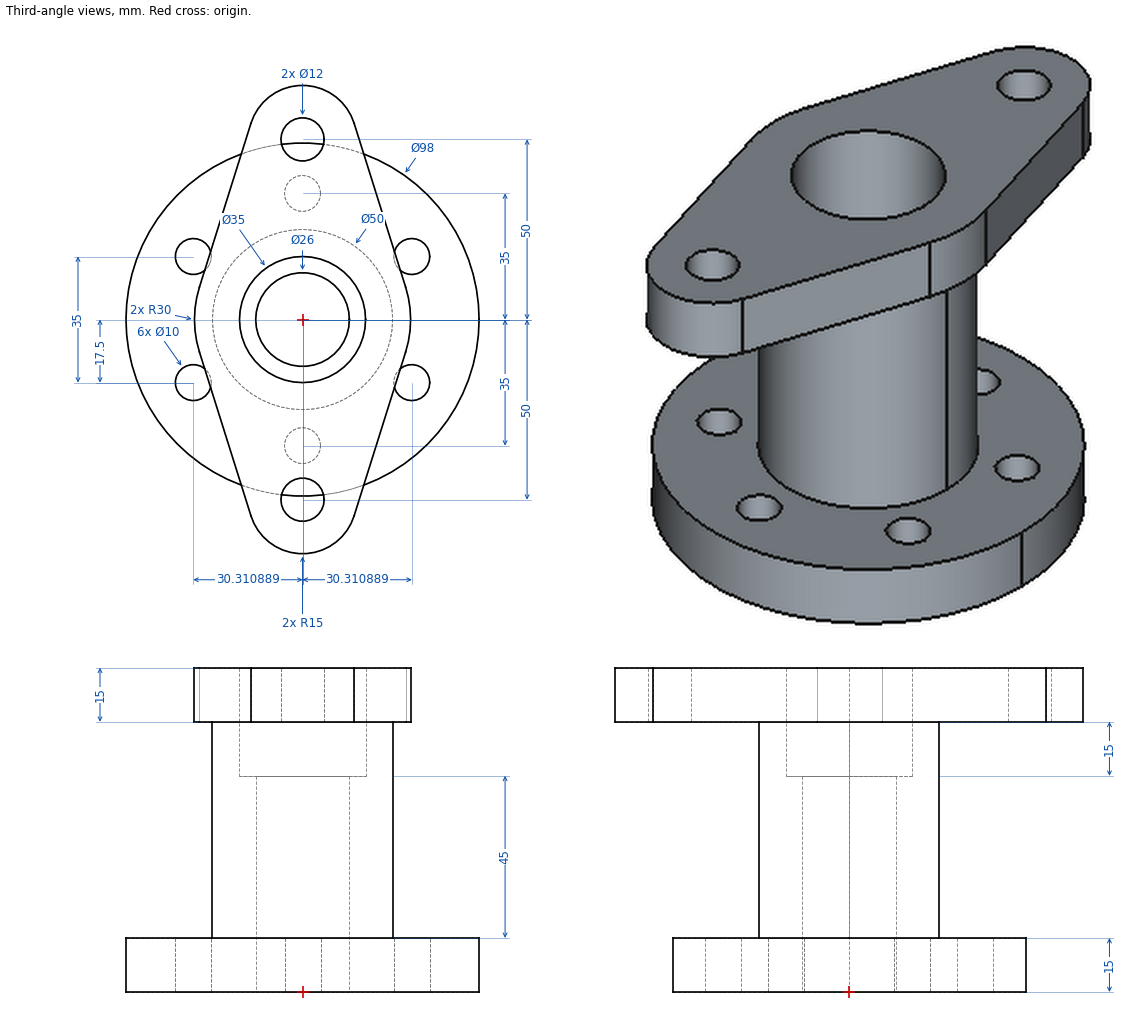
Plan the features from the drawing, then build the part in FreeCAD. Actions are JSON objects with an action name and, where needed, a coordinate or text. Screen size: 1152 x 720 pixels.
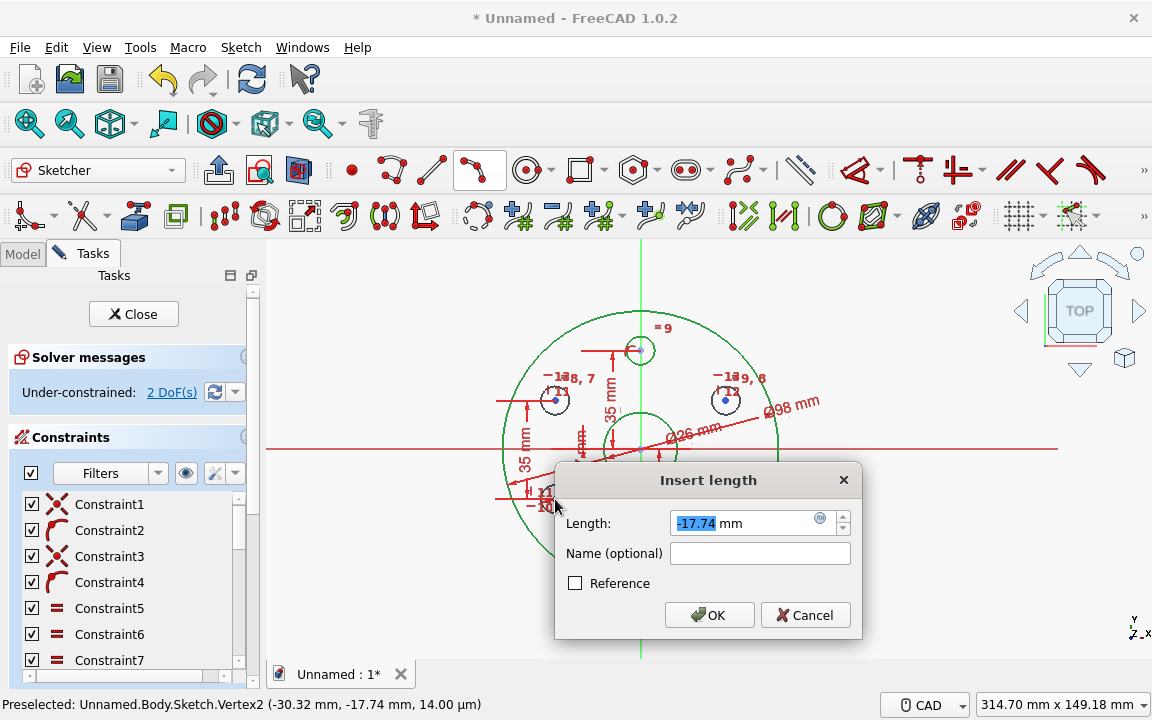
{"action": "type", "text": "-17.5"}
{"action": "key", "text": "Return"}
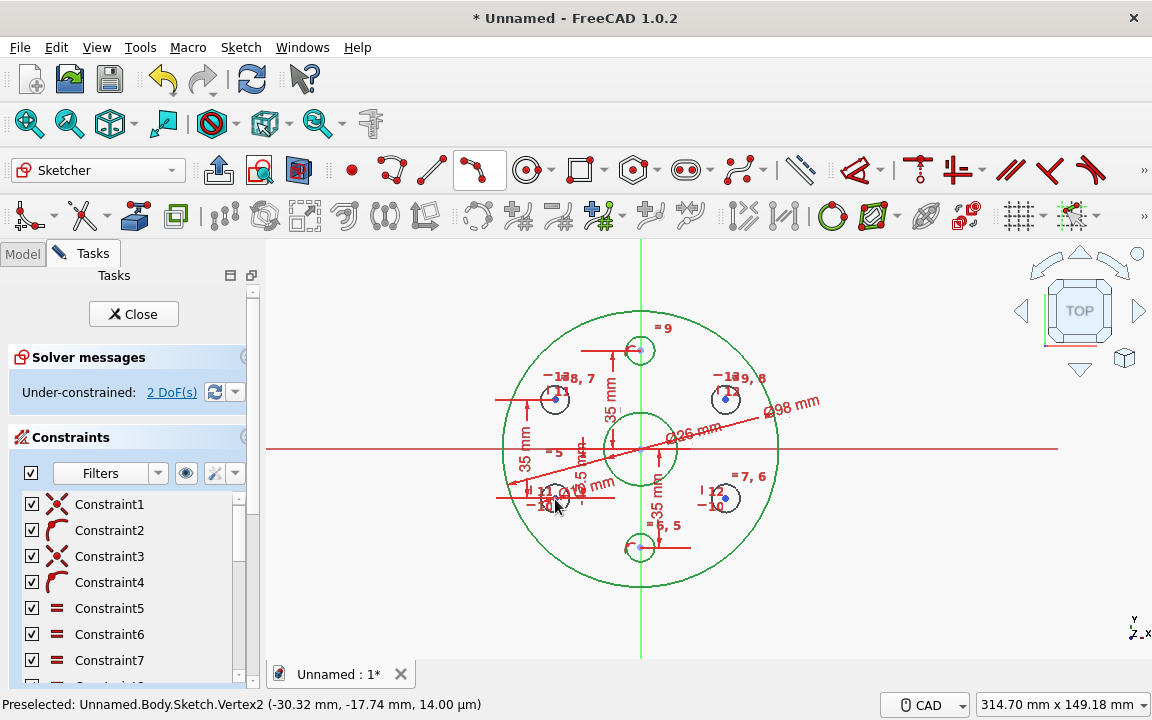
{"action": "left_click", "coordinate": [555, 498]}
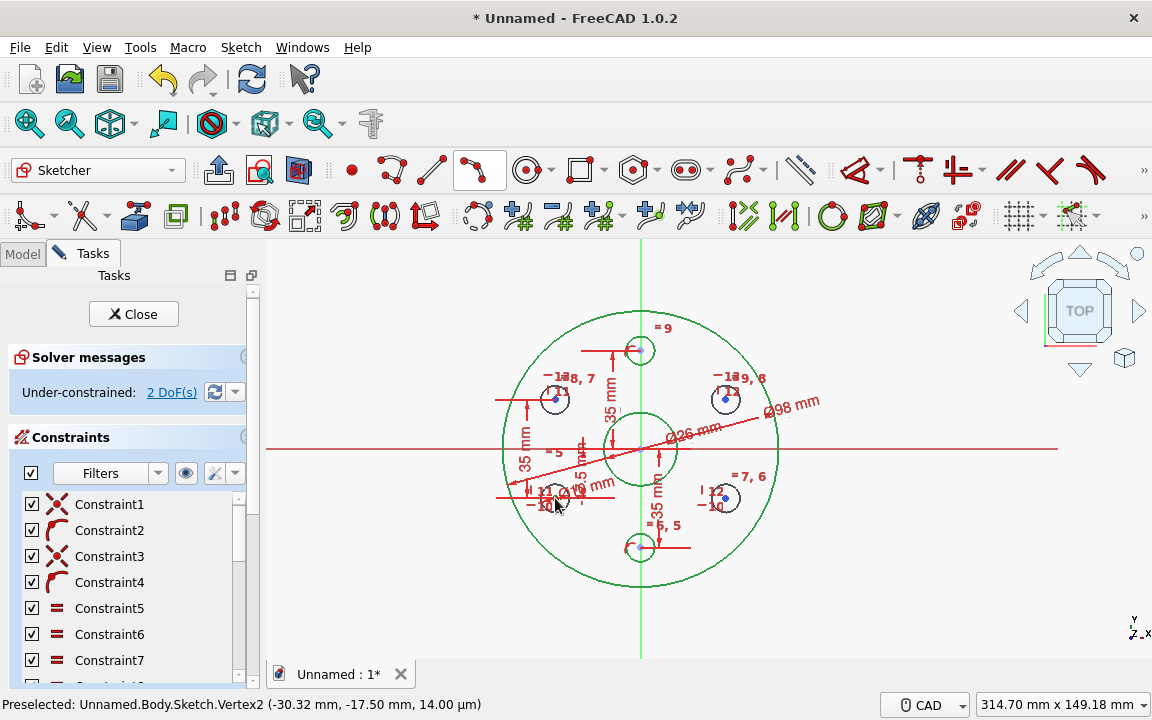
{"action": "key", "text": "l"}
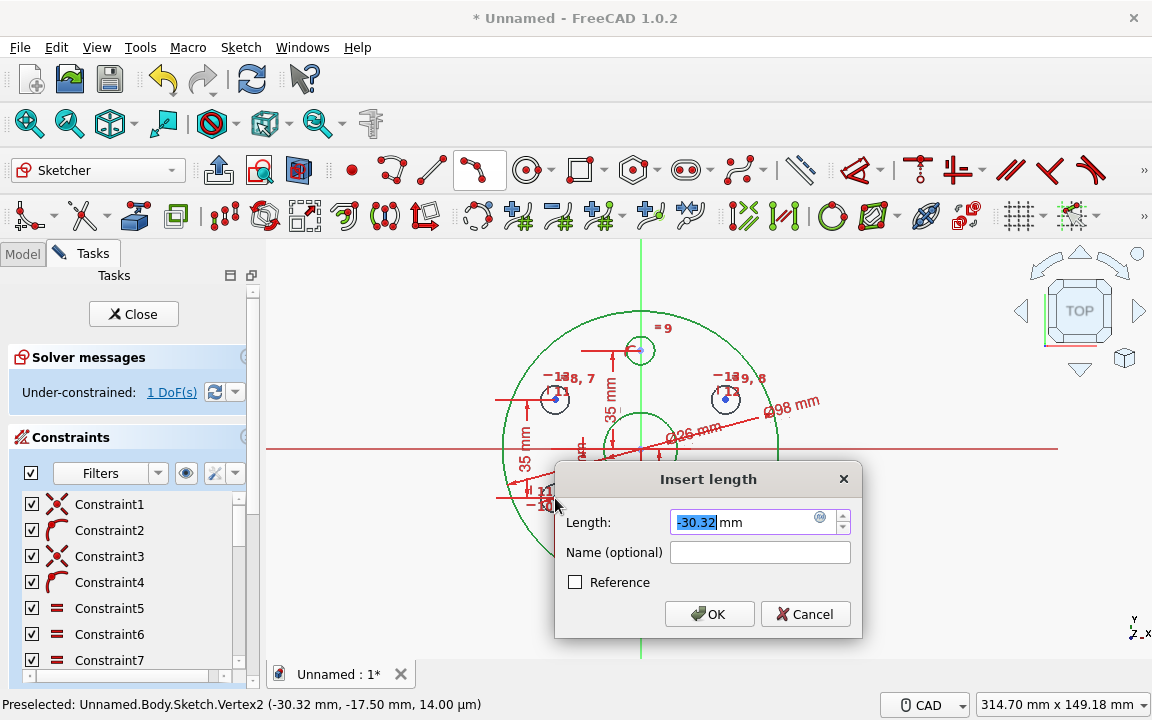
{"action": "type", "text": "-30.310889"}
{"action": "key", "text": "Return"}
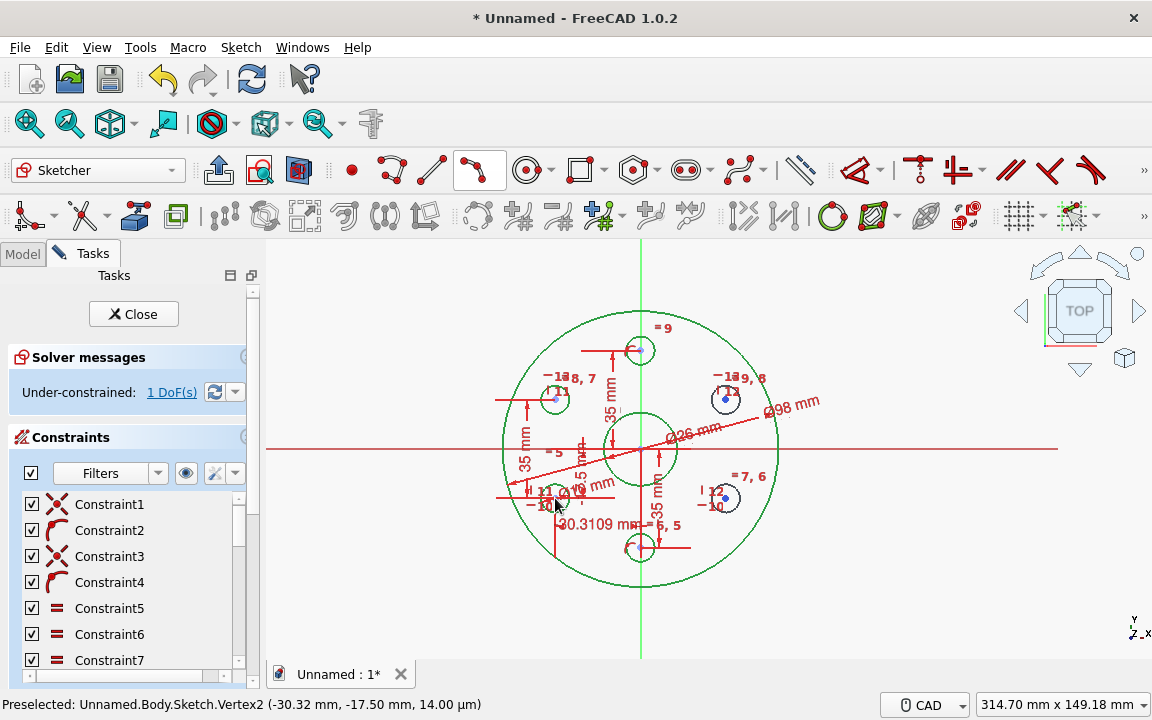
{"action": "left_click", "coordinate": [726, 498]}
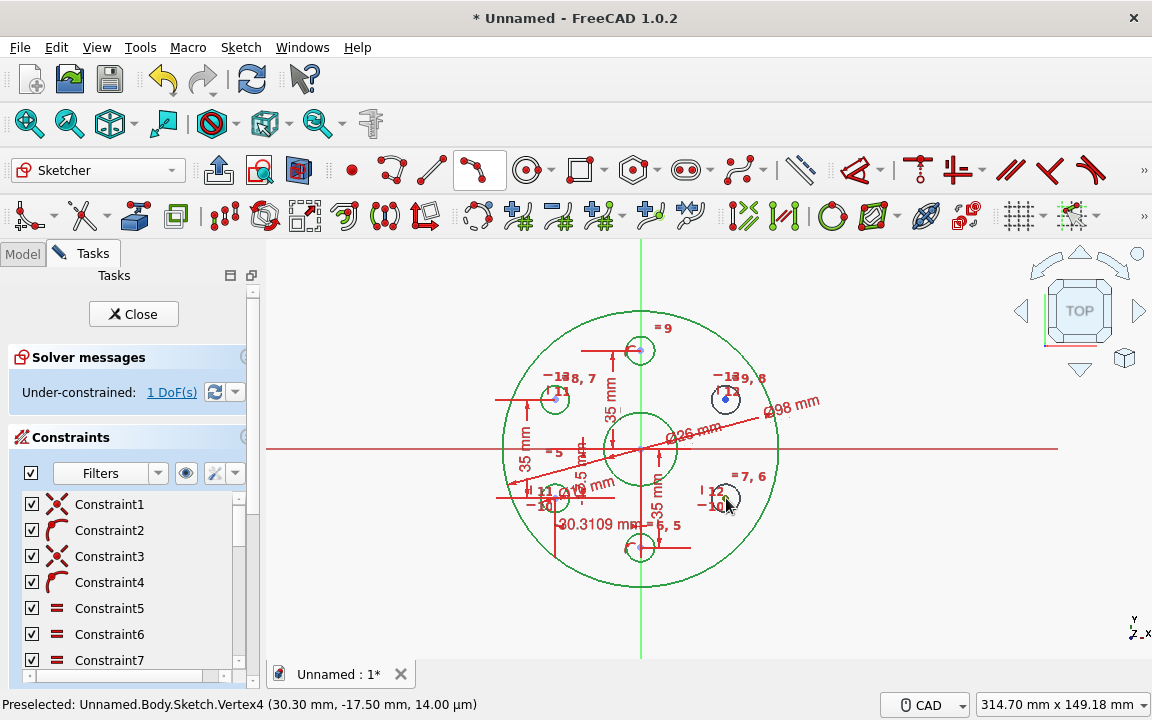
{"action": "key", "text": "l"}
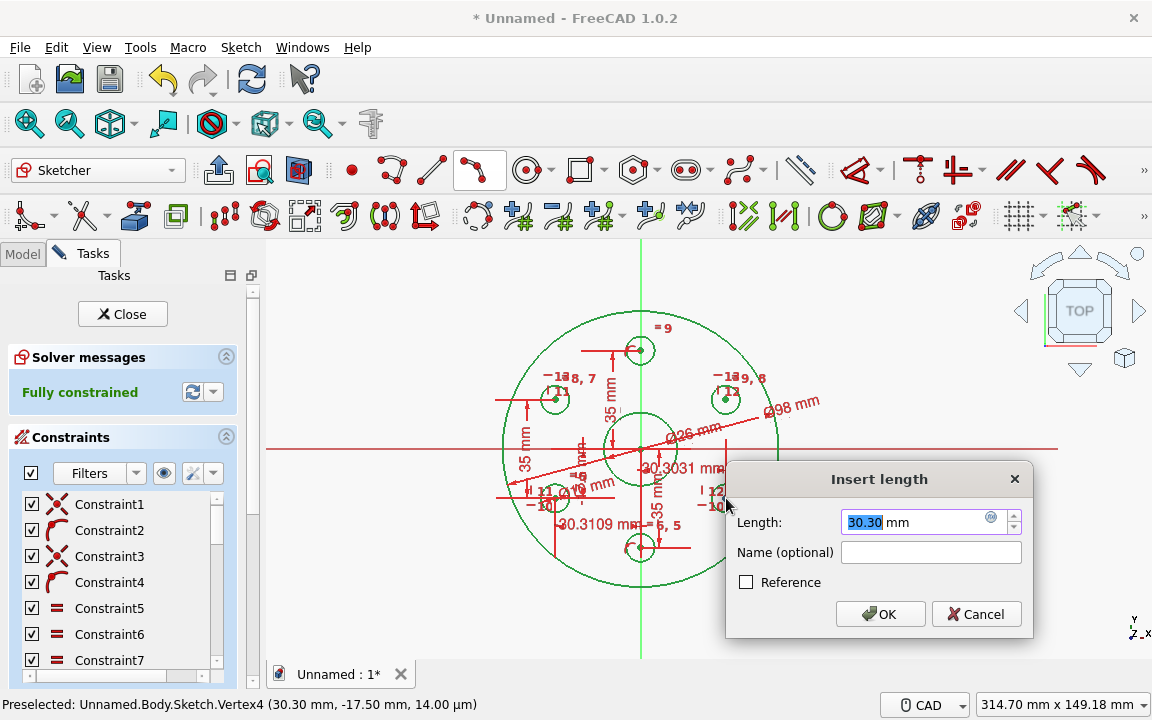
{"action": "type", "text": "30.310889"}
{"action": "key", "text": "Return"}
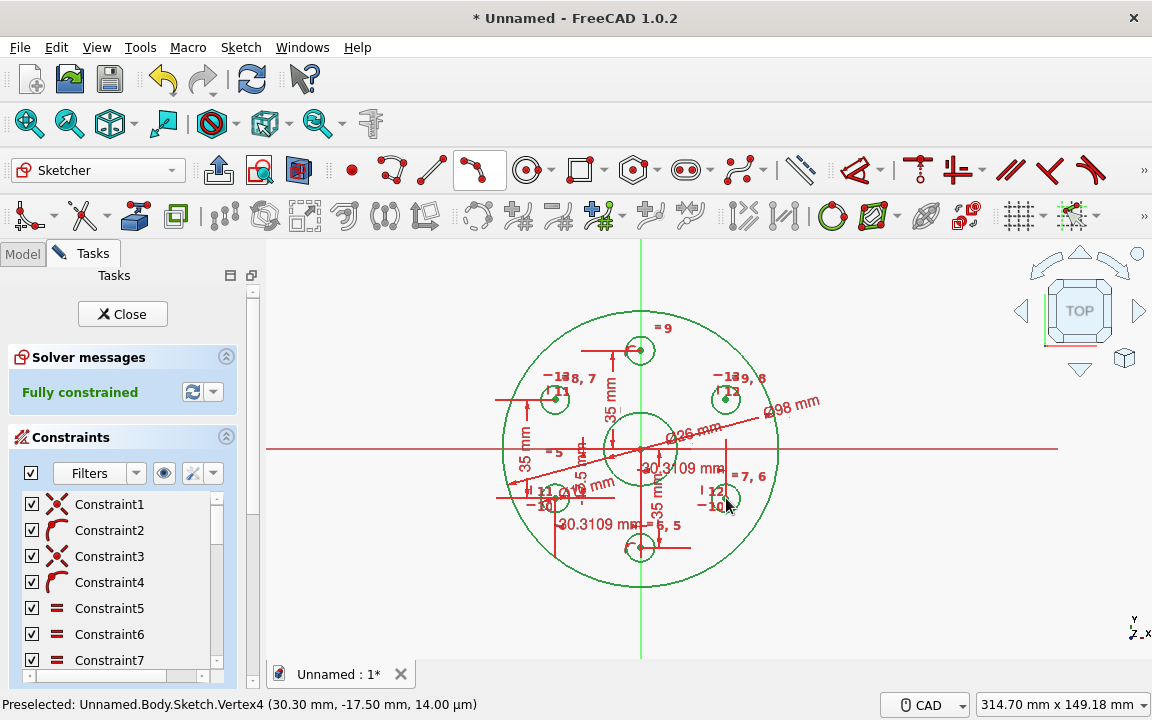
{"action": "left_click", "coordinate": [123, 314]}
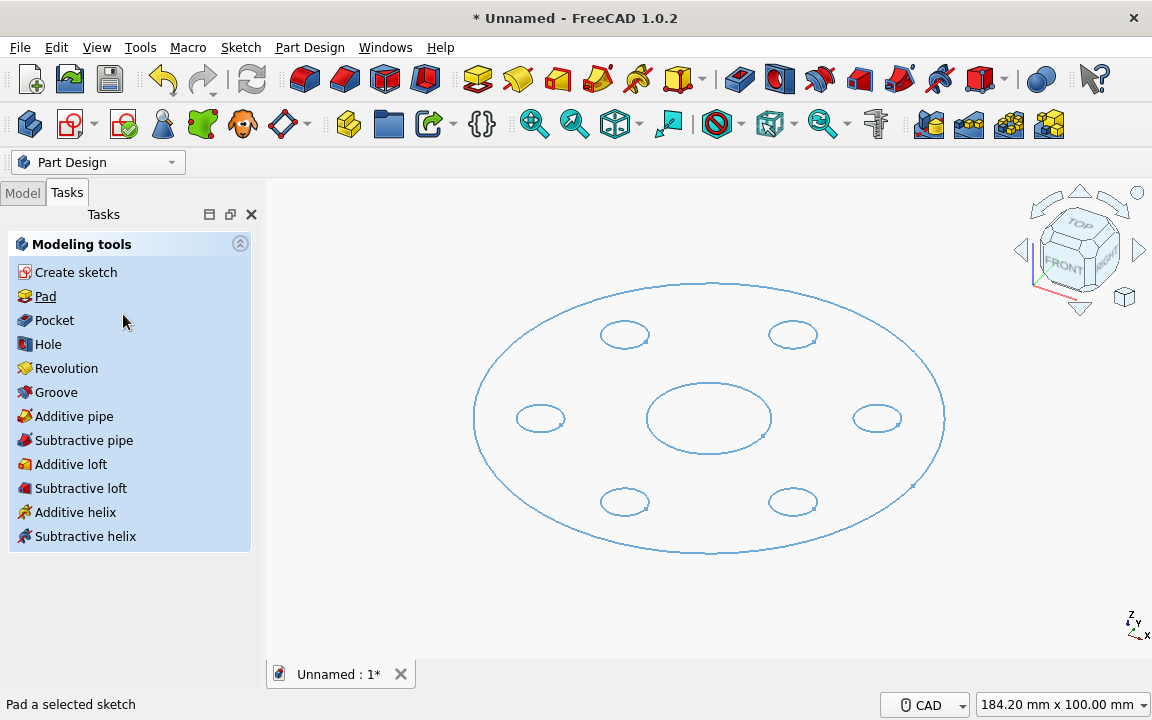
{"action": "left_click", "coordinate": [478, 80]}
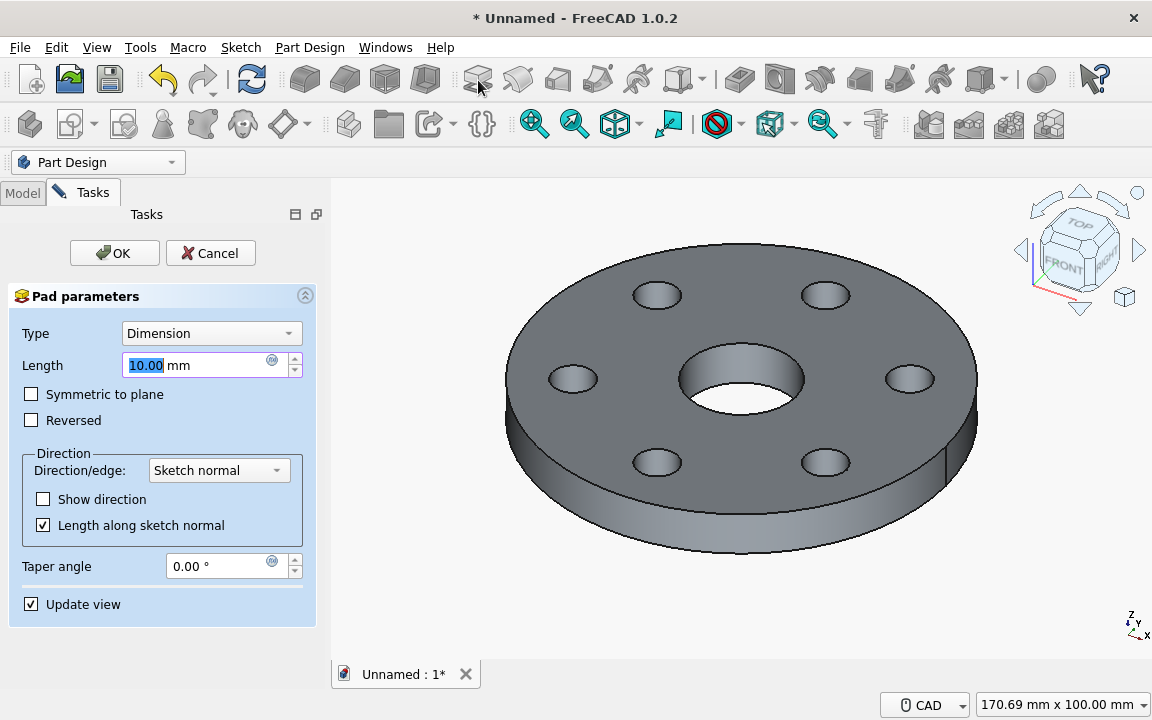
{"action": "type", "text": "15"}
{"action": "key", "text": "Tab"}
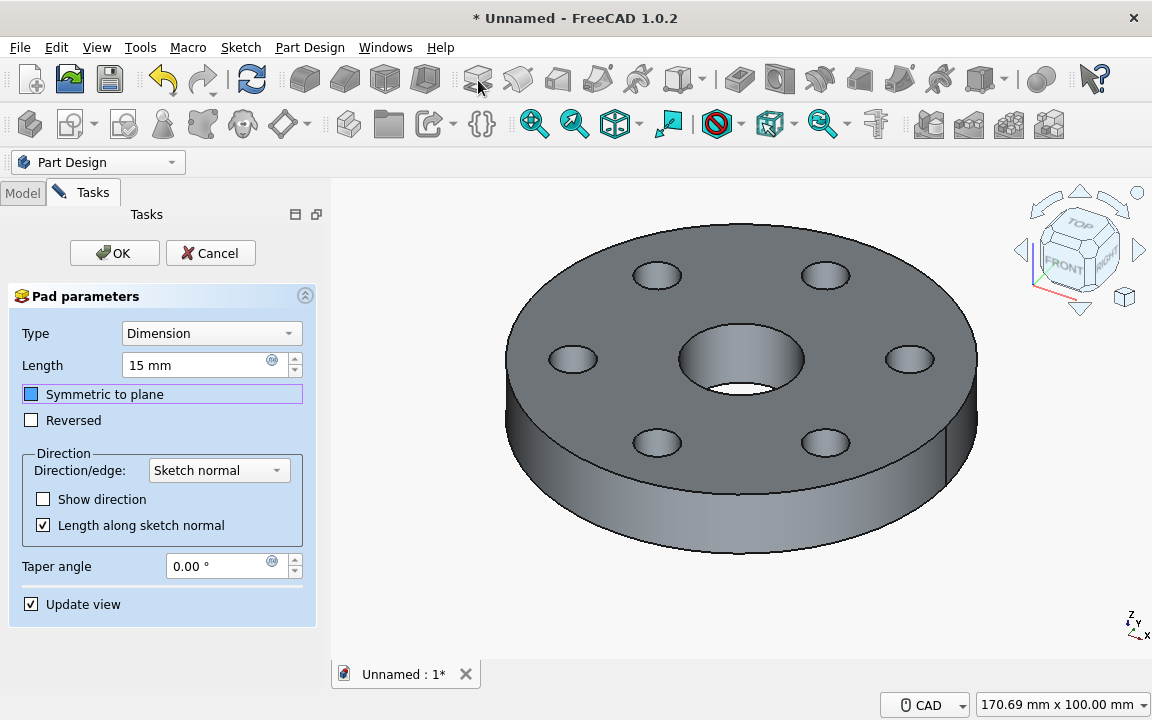
{"action": "left_click", "coordinate": [115, 253]}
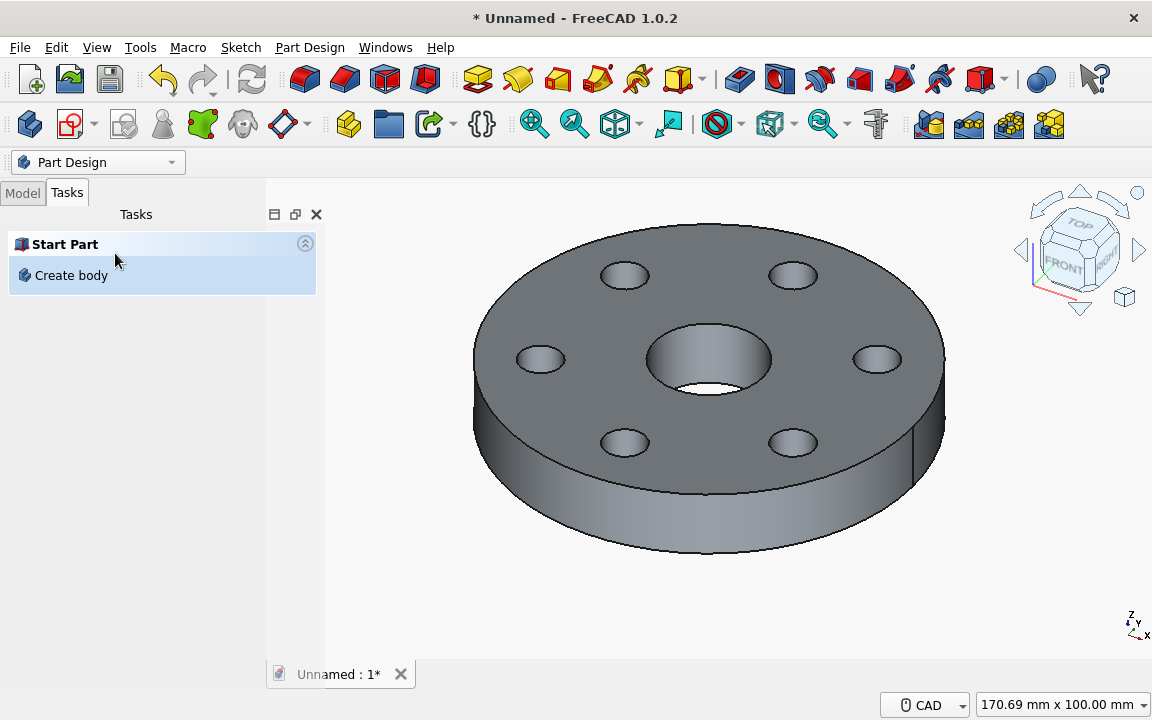
{"action": "key", "text": "v f"}